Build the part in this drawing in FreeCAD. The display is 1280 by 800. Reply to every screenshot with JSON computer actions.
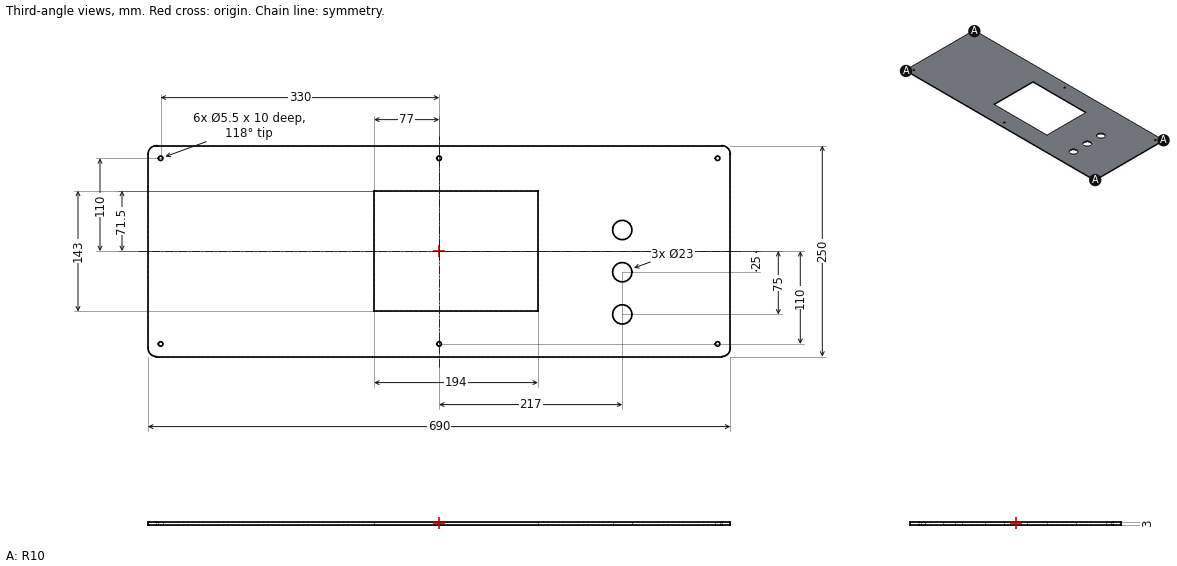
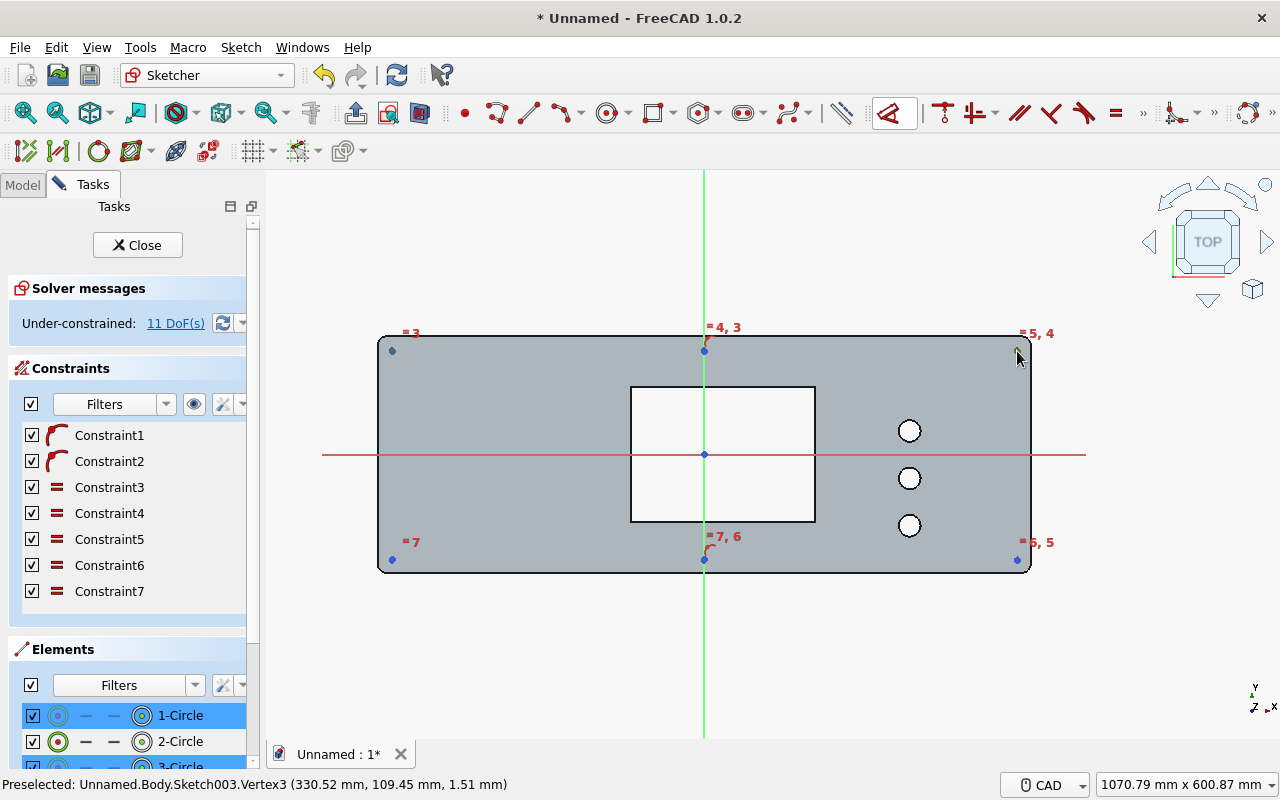
{"action": "left_click", "coordinate": [704, 674]}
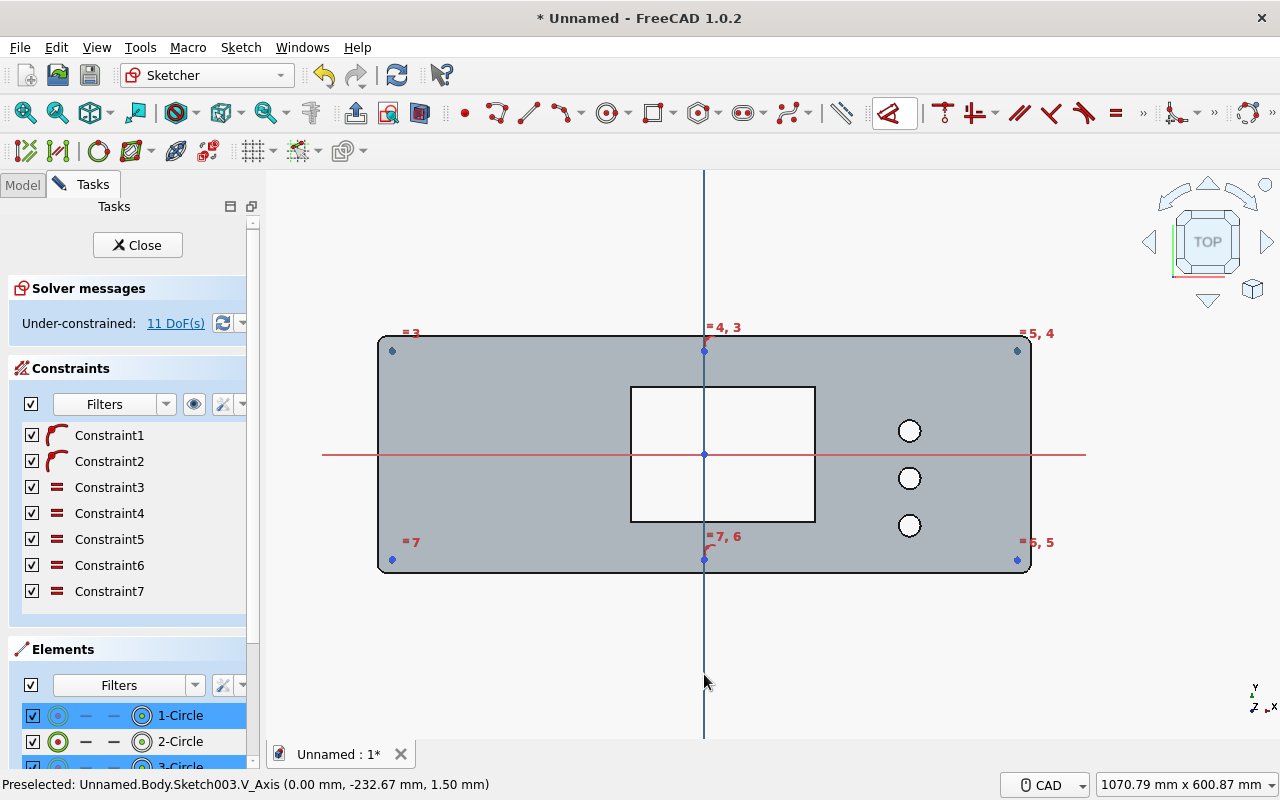
{"action": "key", "text": "s"}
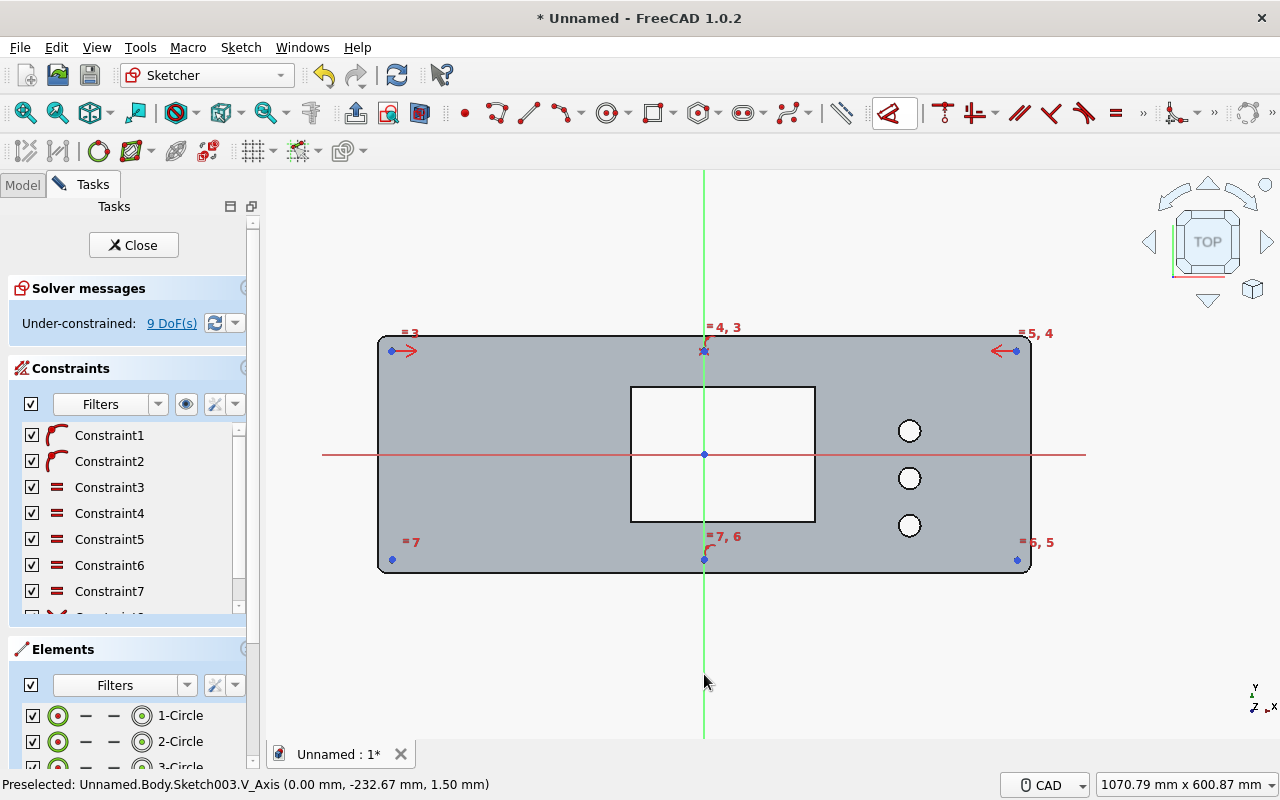
{"action": "left_click", "coordinate": [1016, 351]}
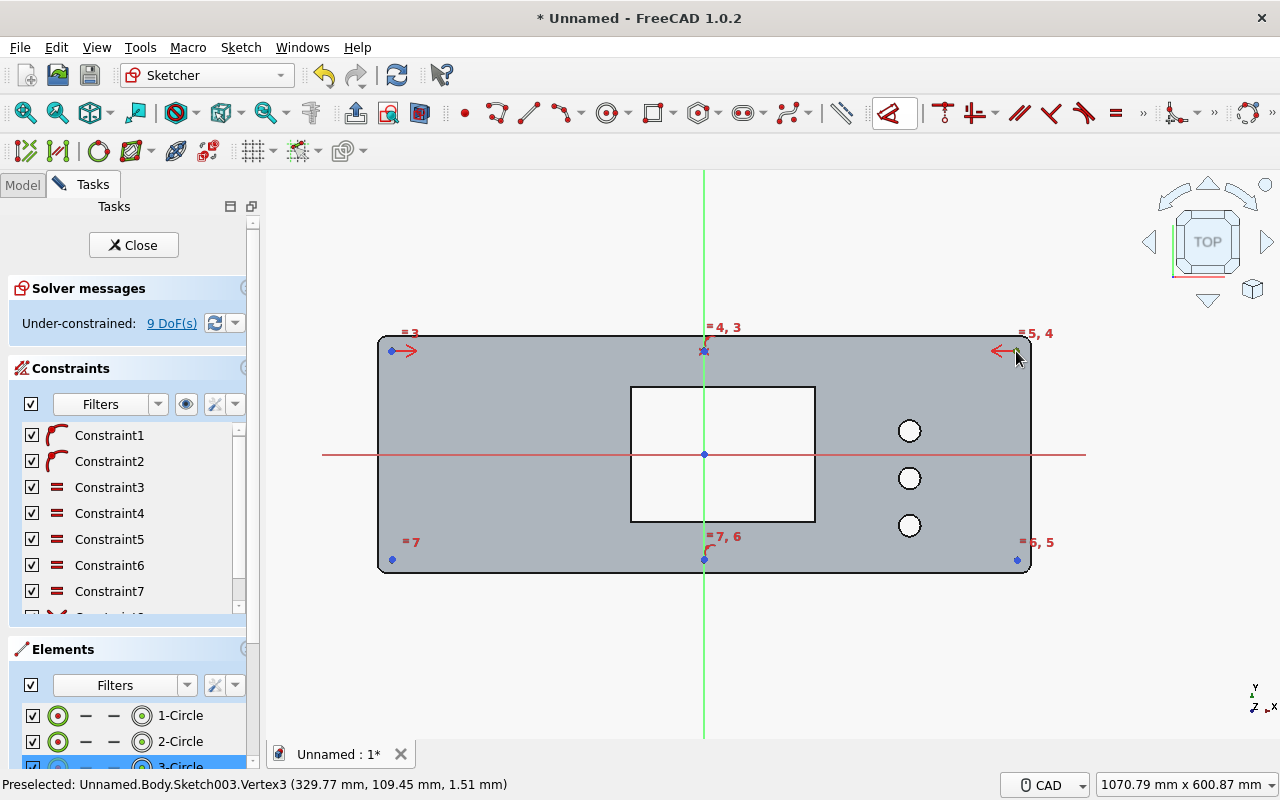
{"action": "left_click", "coordinate": [1017, 560]}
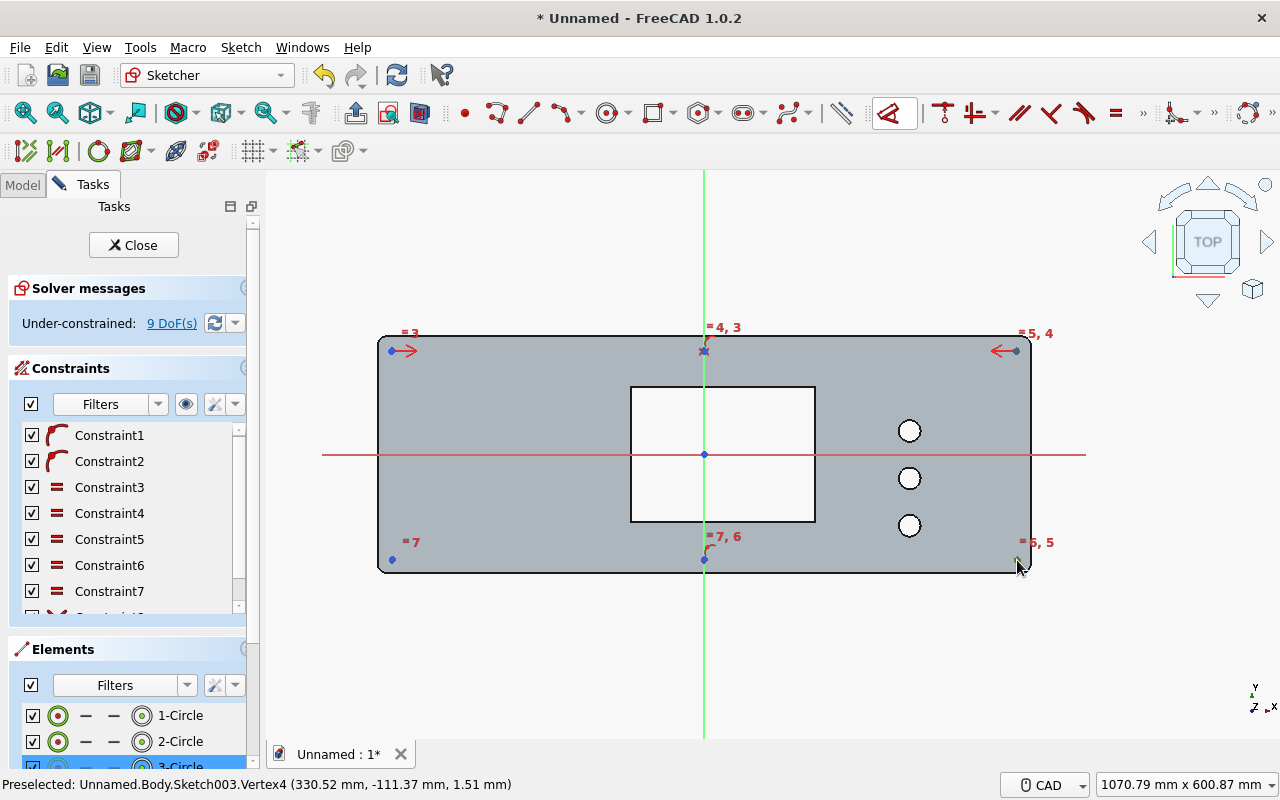
{"action": "left_click", "coordinate": [353, 455]}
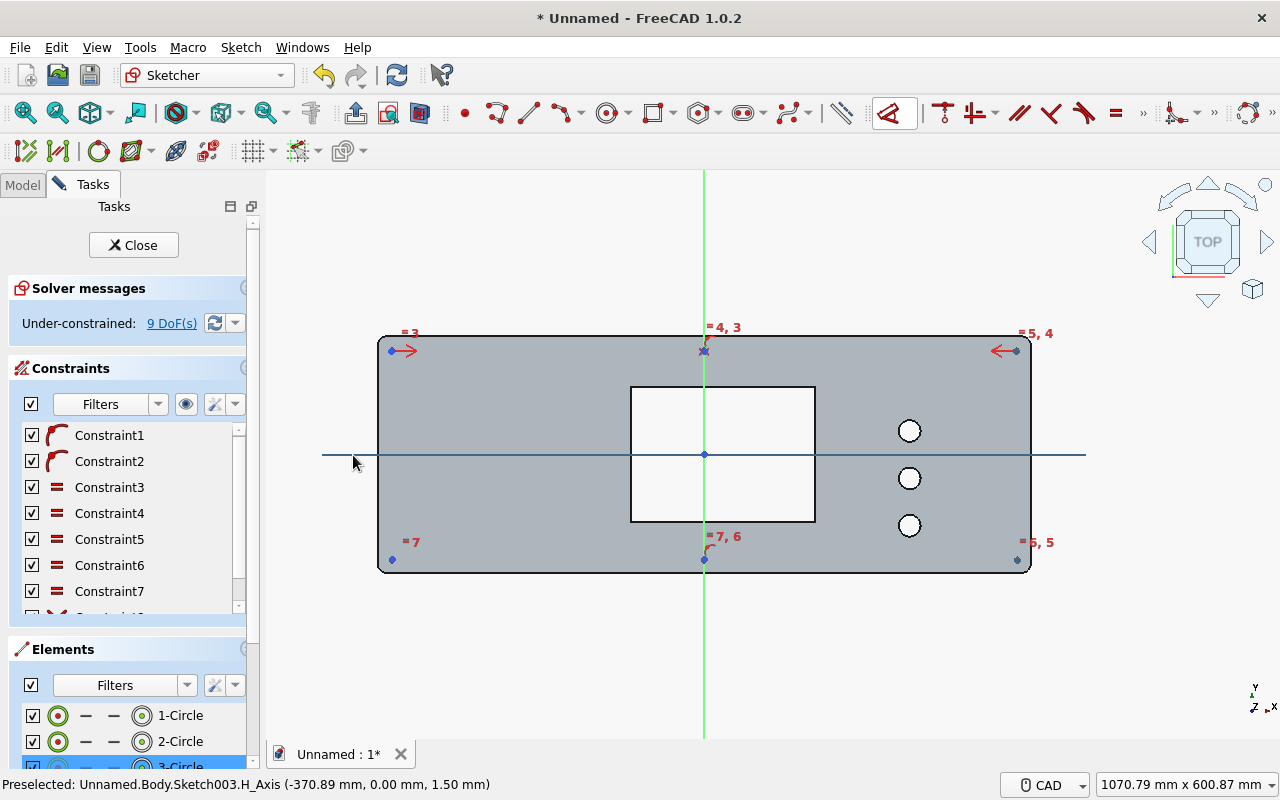
{"action": "key", "text": "s"}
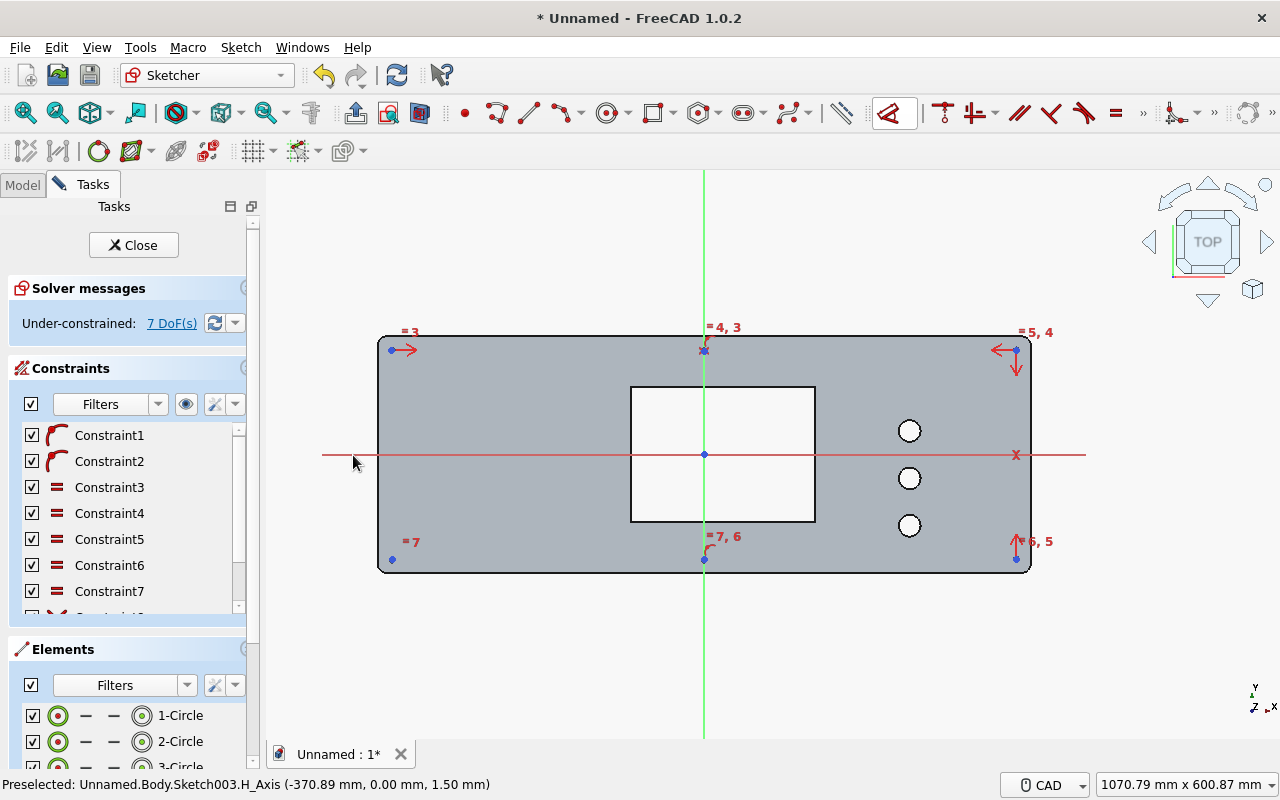
{"action": "left_click", "coordinate": [392, 350]}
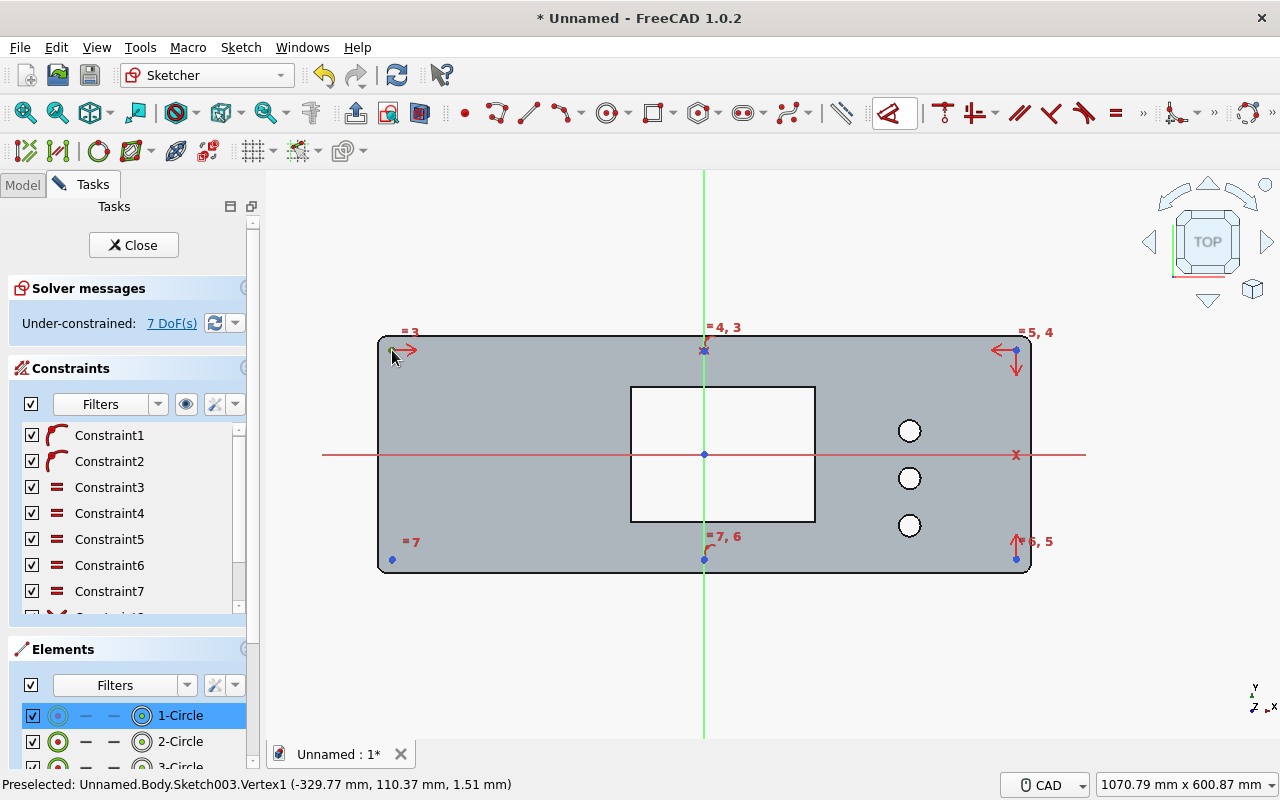
{"action": "left_click", "coordinate": [392, 560]}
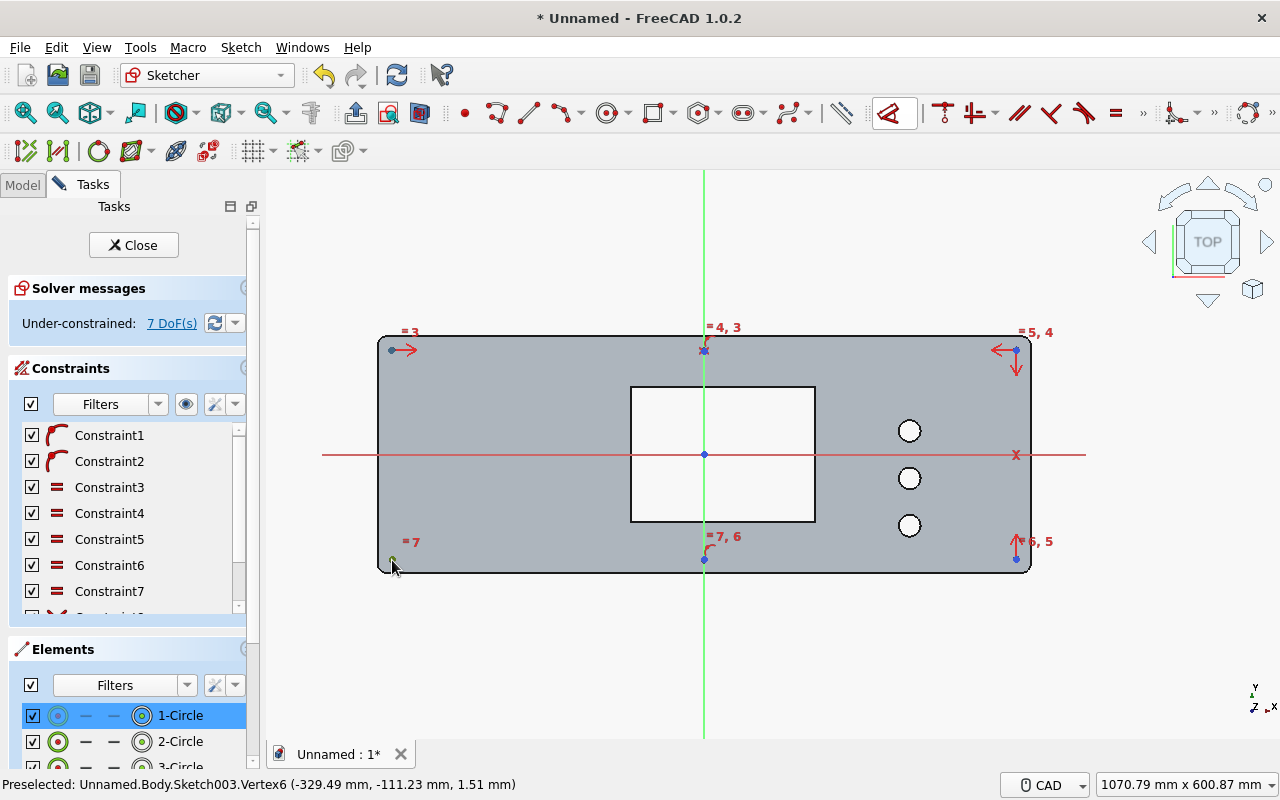
{"action": "left_click", "coordinate": [353, 455]}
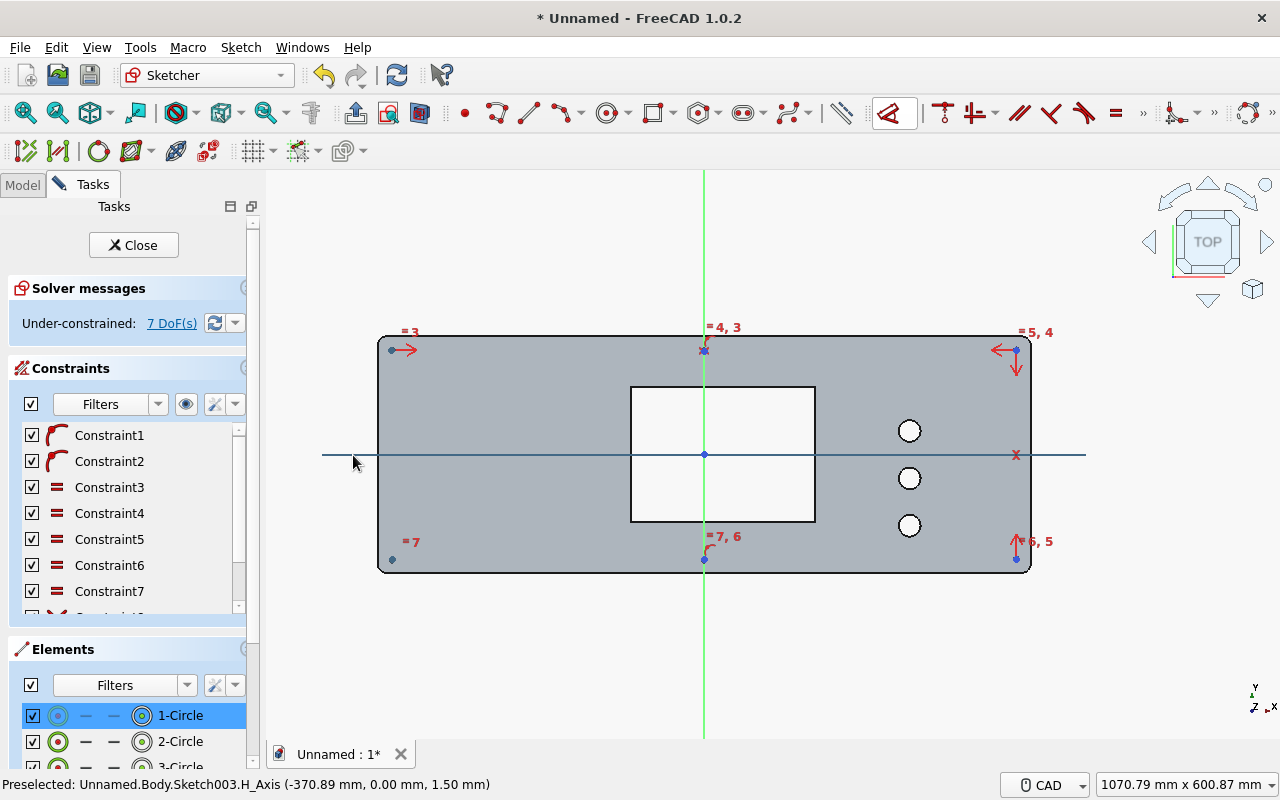
{"action": "key", "text": "s"}